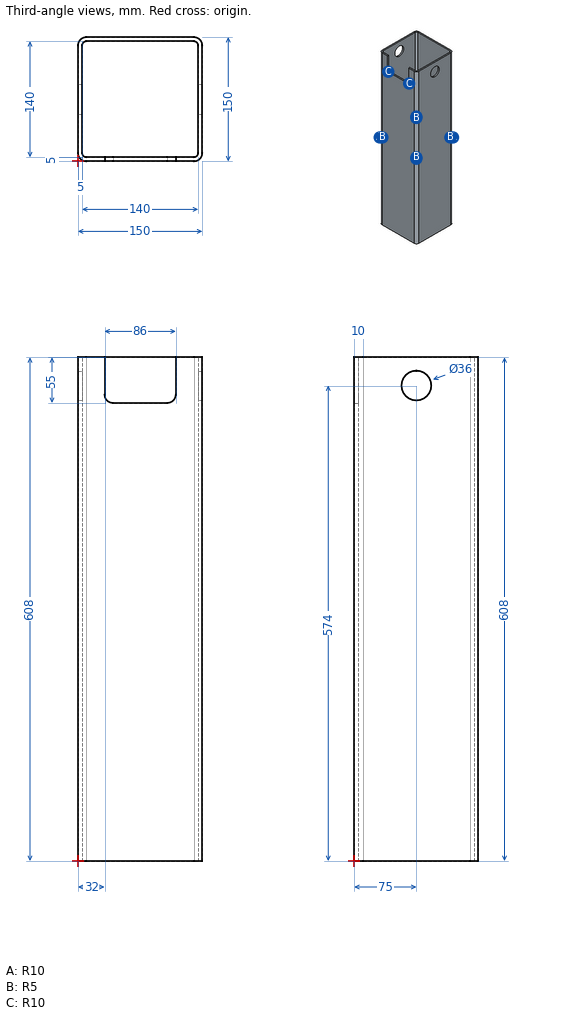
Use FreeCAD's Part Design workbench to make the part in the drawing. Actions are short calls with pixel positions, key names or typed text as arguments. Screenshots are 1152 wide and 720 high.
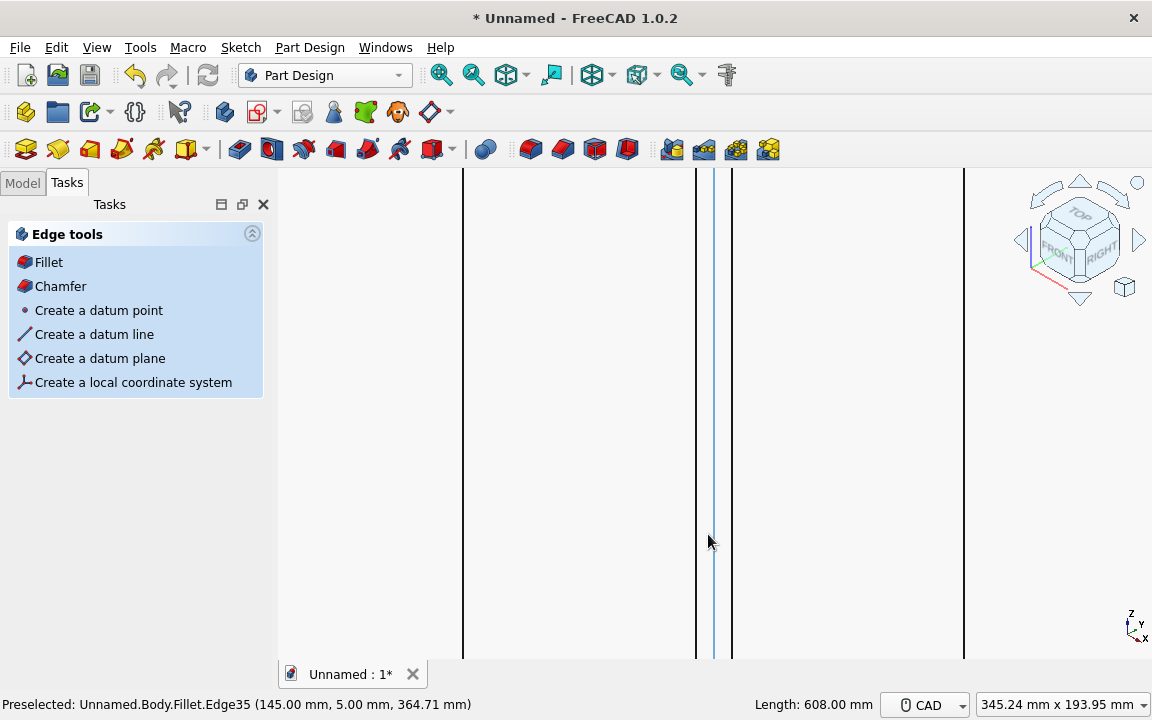
key(v)
key(f)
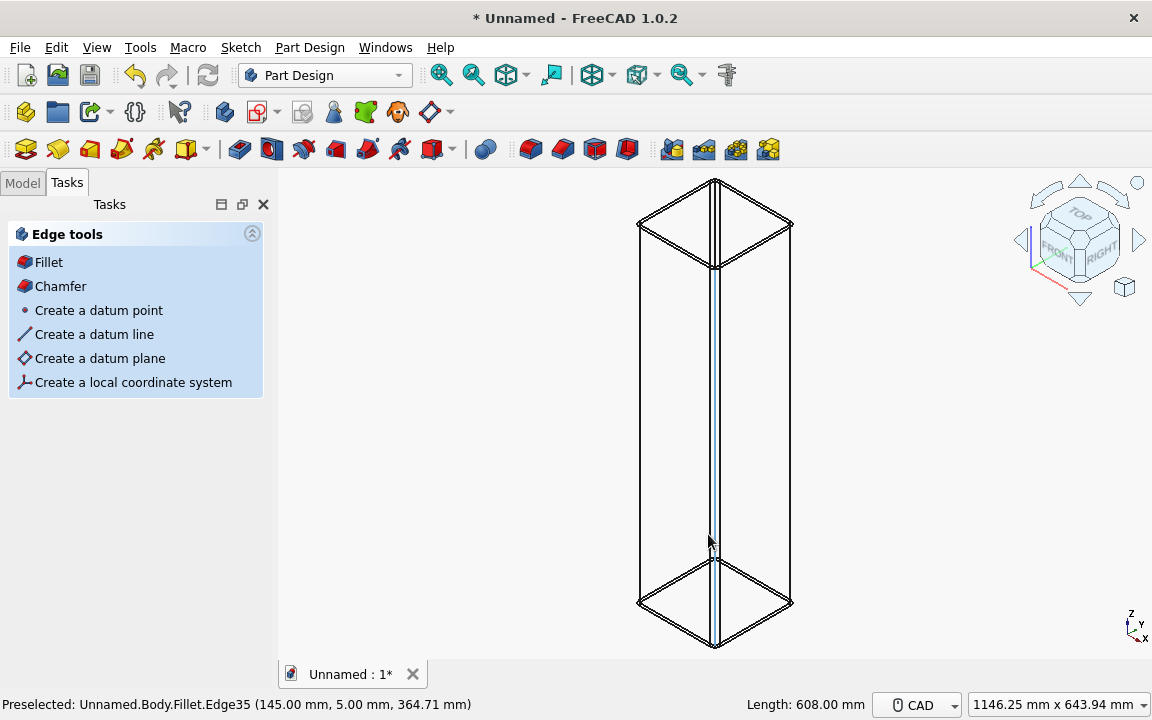
key(2)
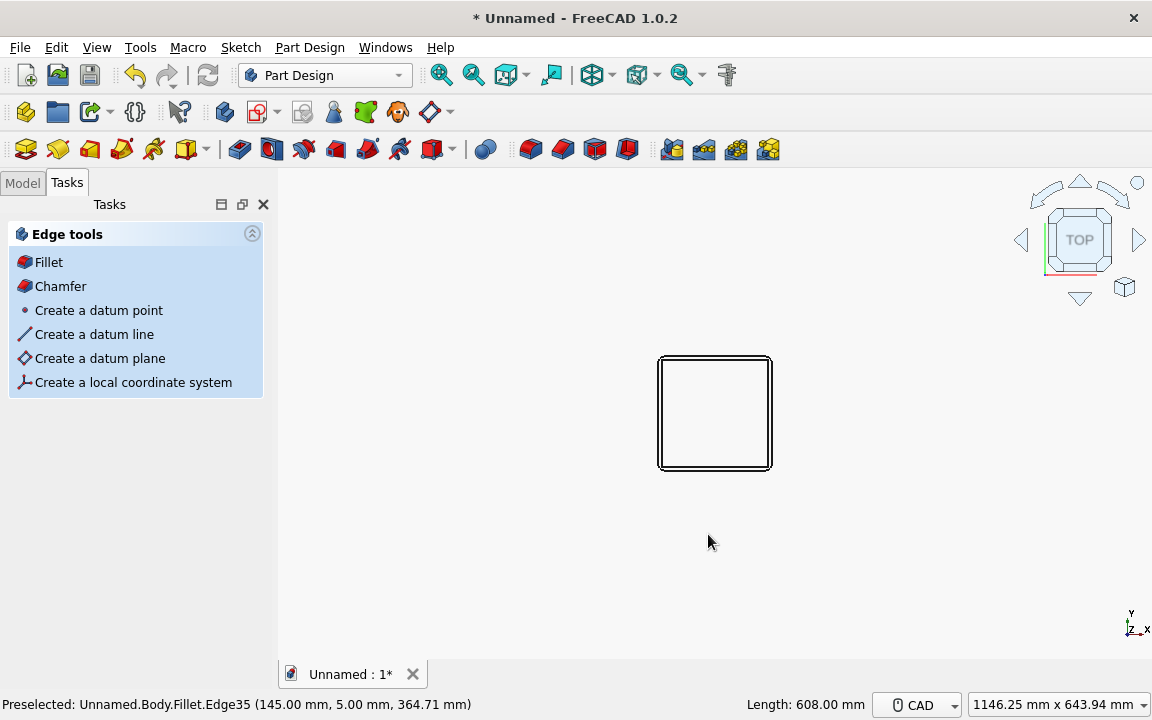
key(v)
key(f)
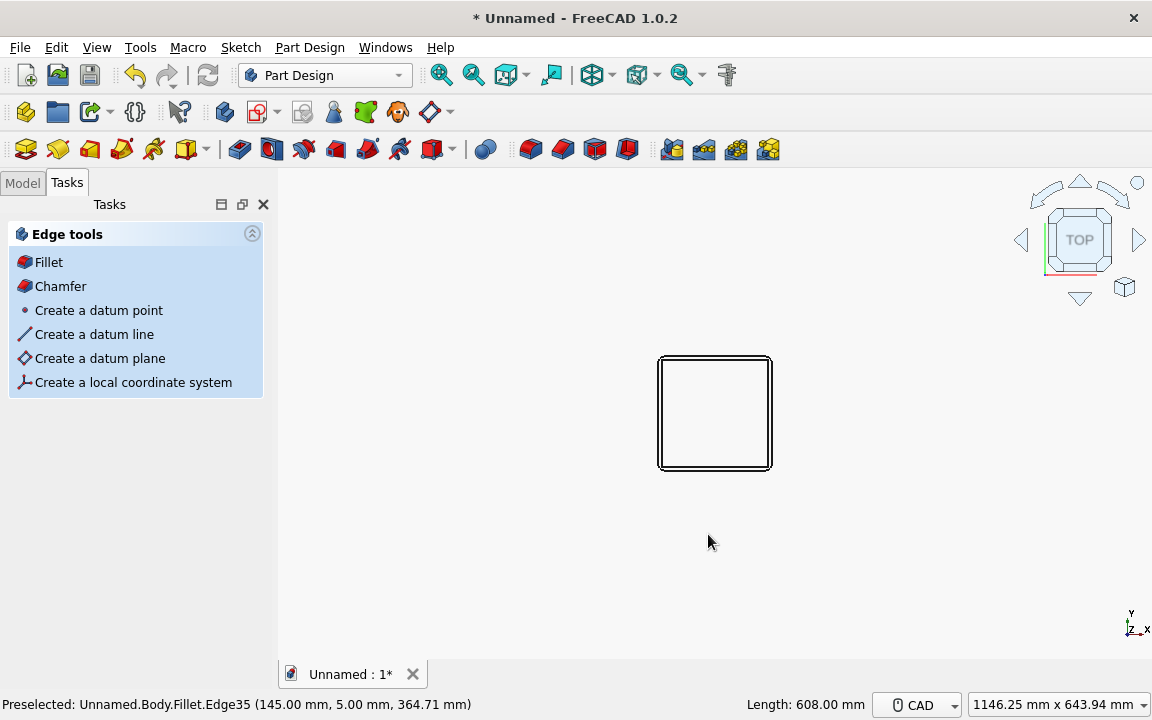
scroll(662, 359, up, 6)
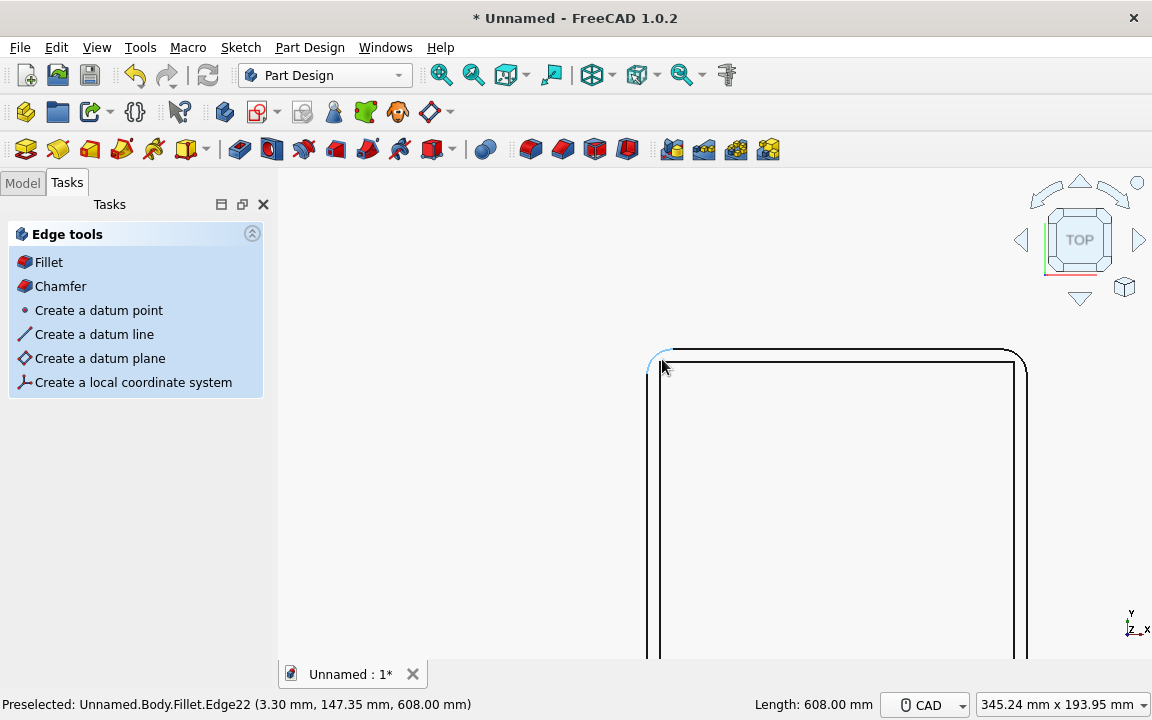
click(442, 76)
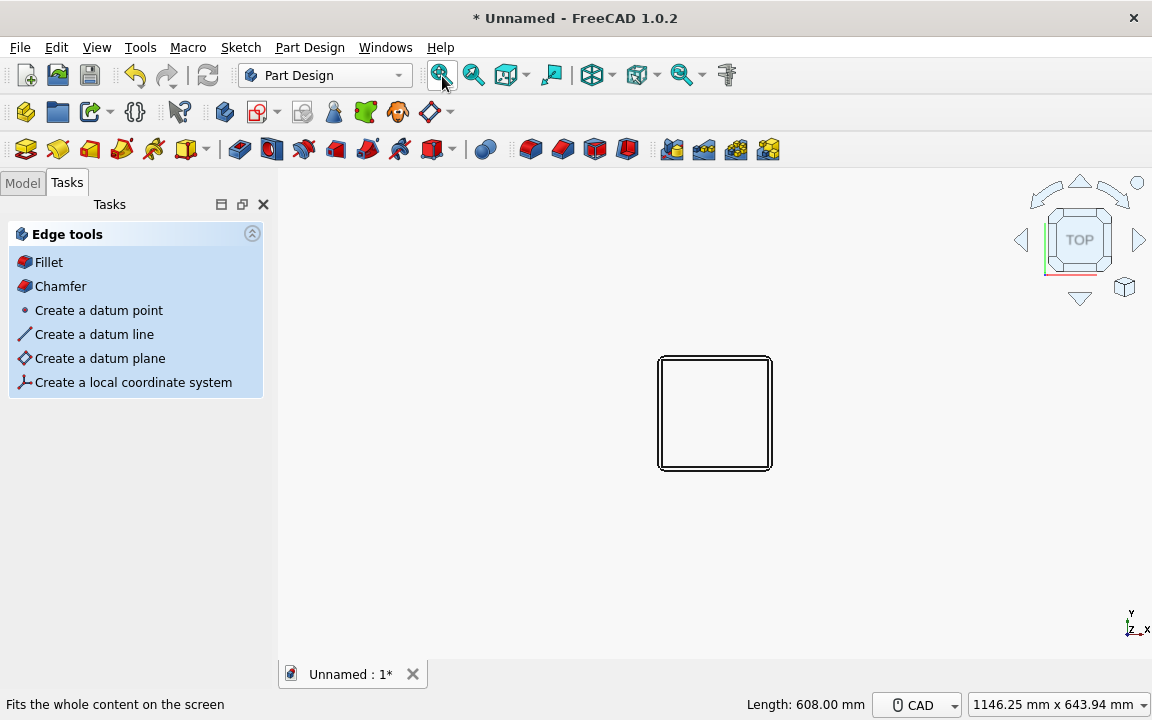
key(1)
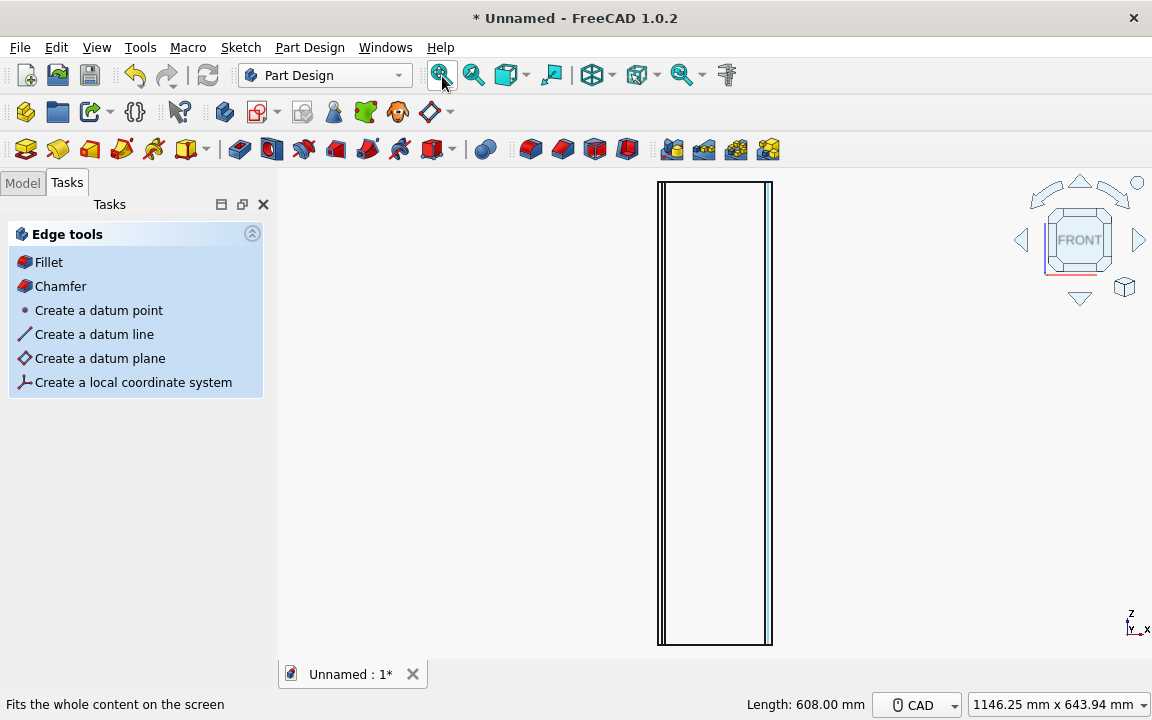
scroll(662, 413, up, 6)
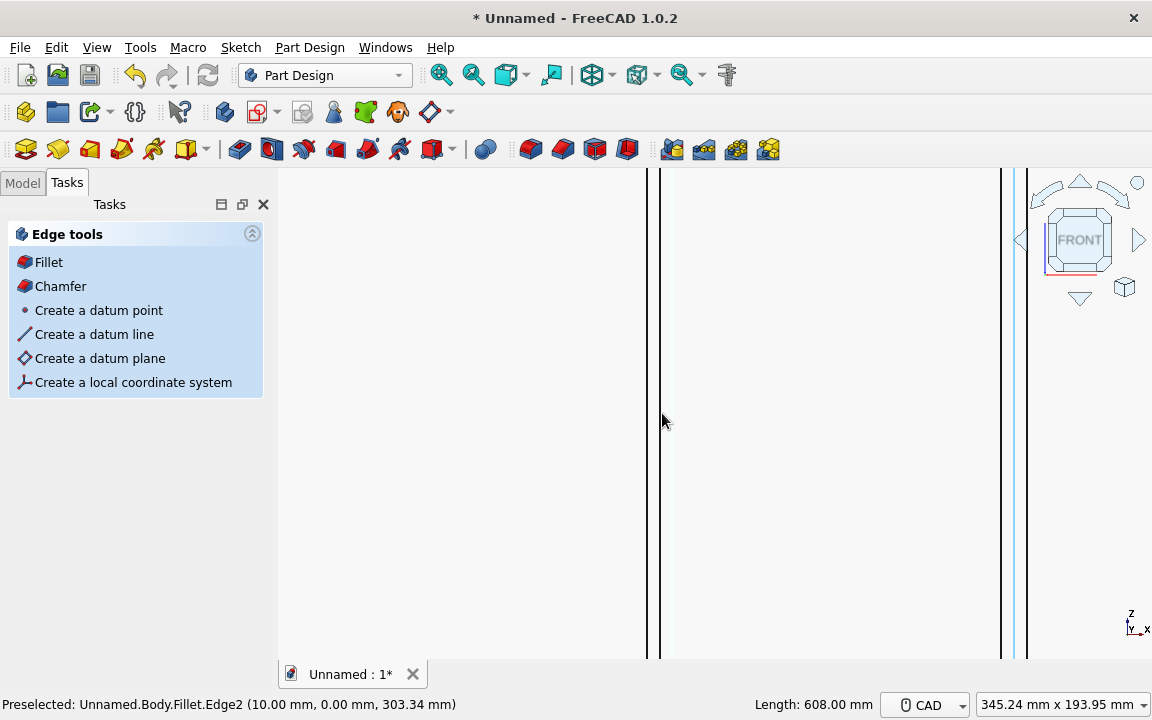
click(660, 413, ctrl)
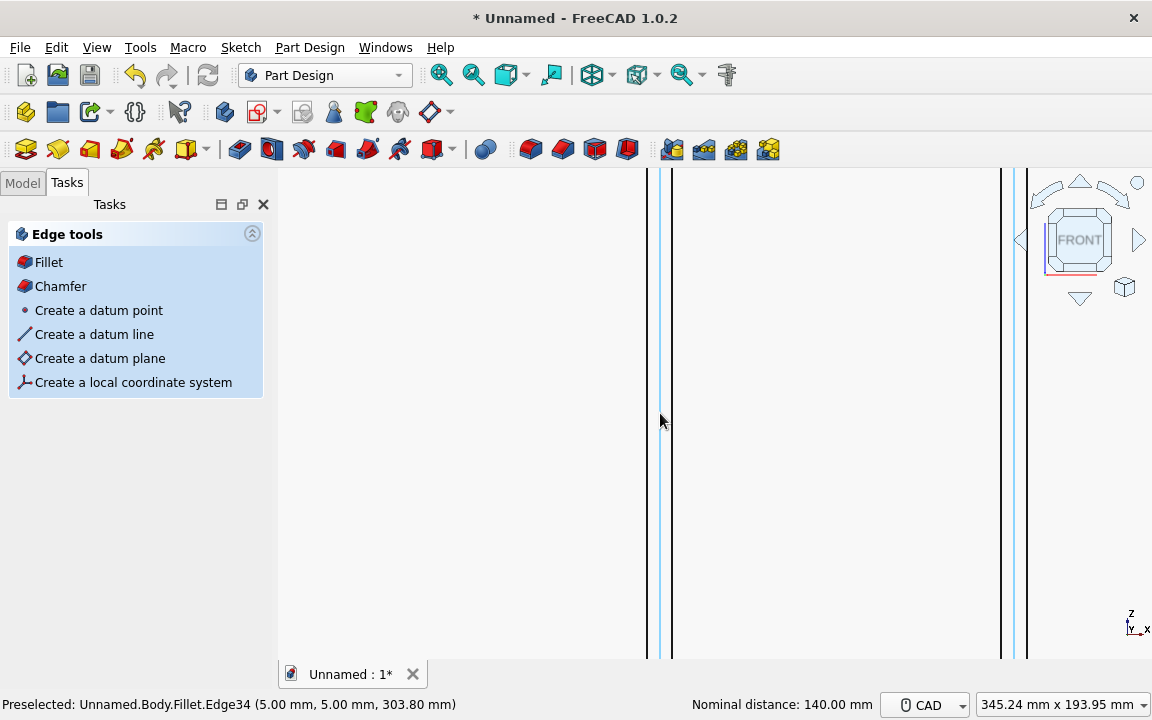
key(v)
key(f)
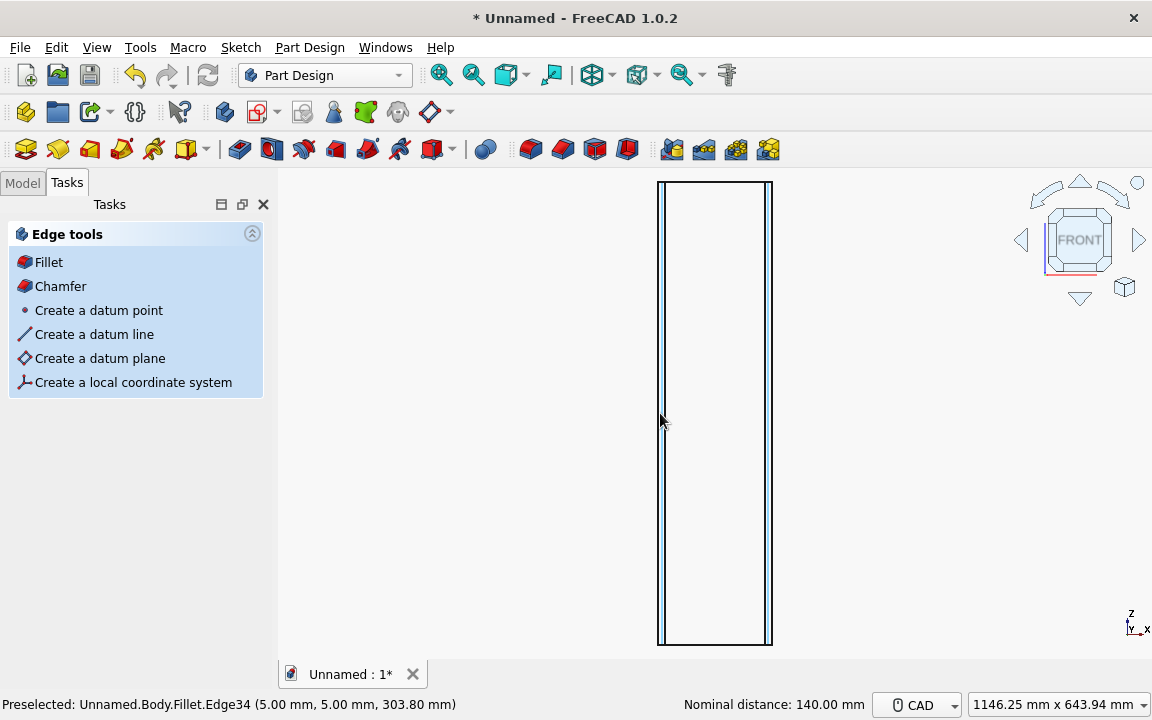
key(3)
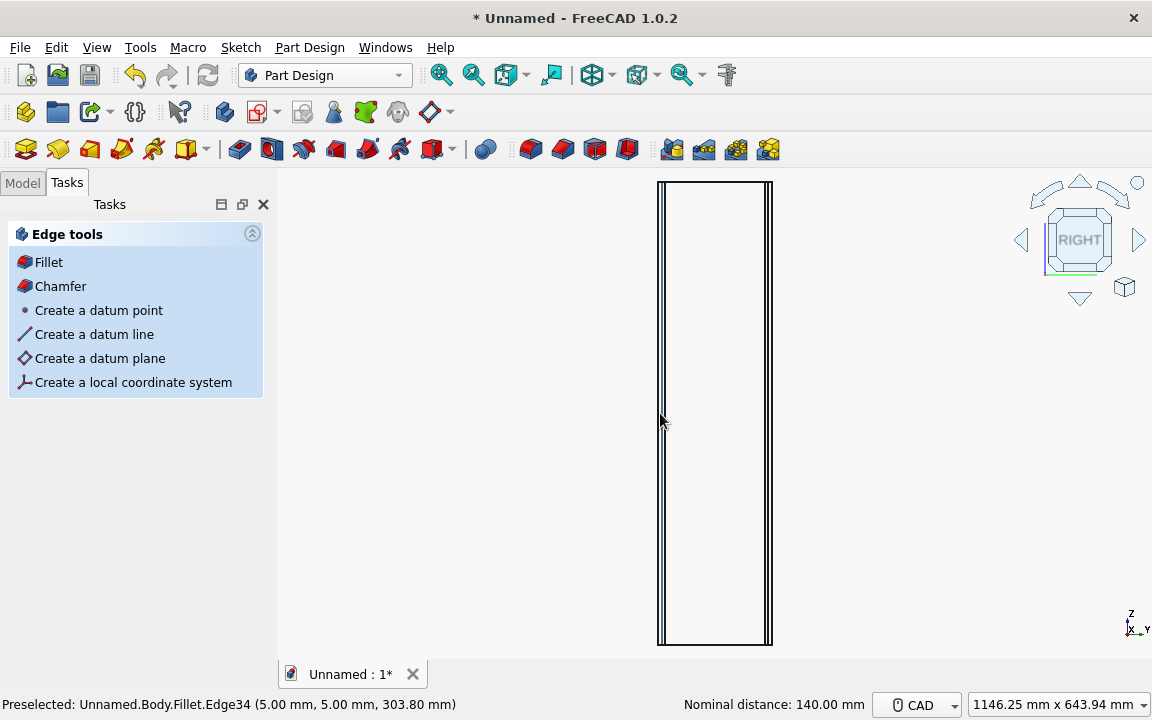
scroll(768, 412, up, 6)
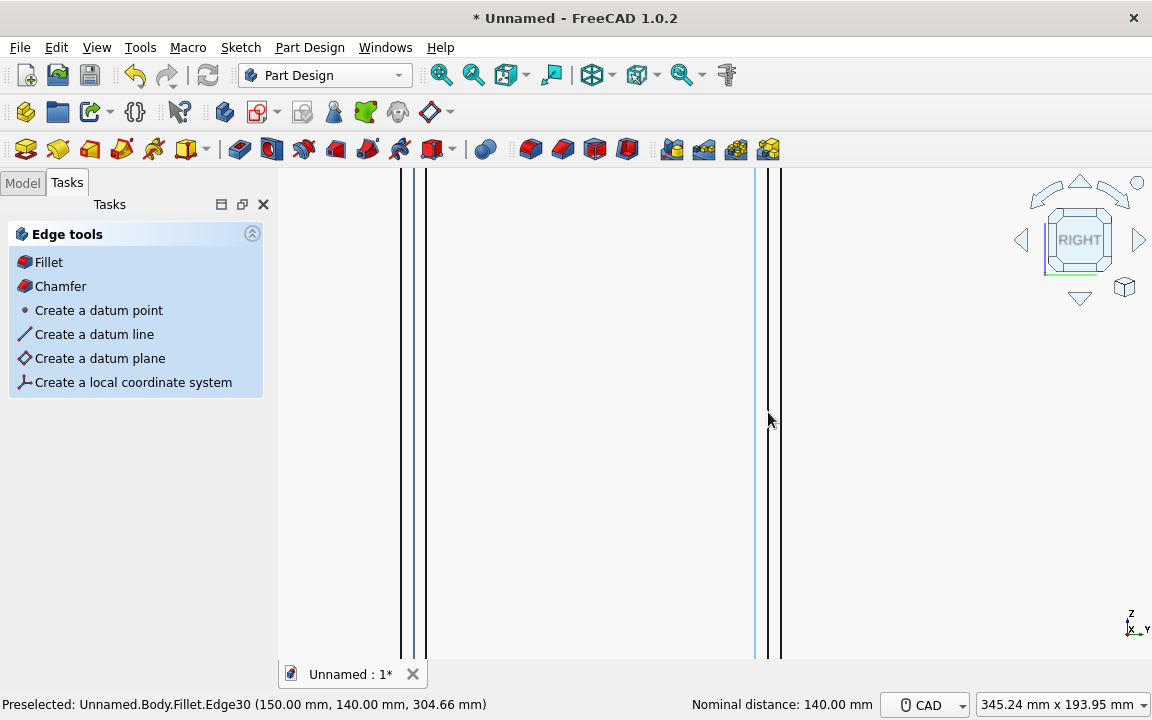
click(768, 415, ctrl)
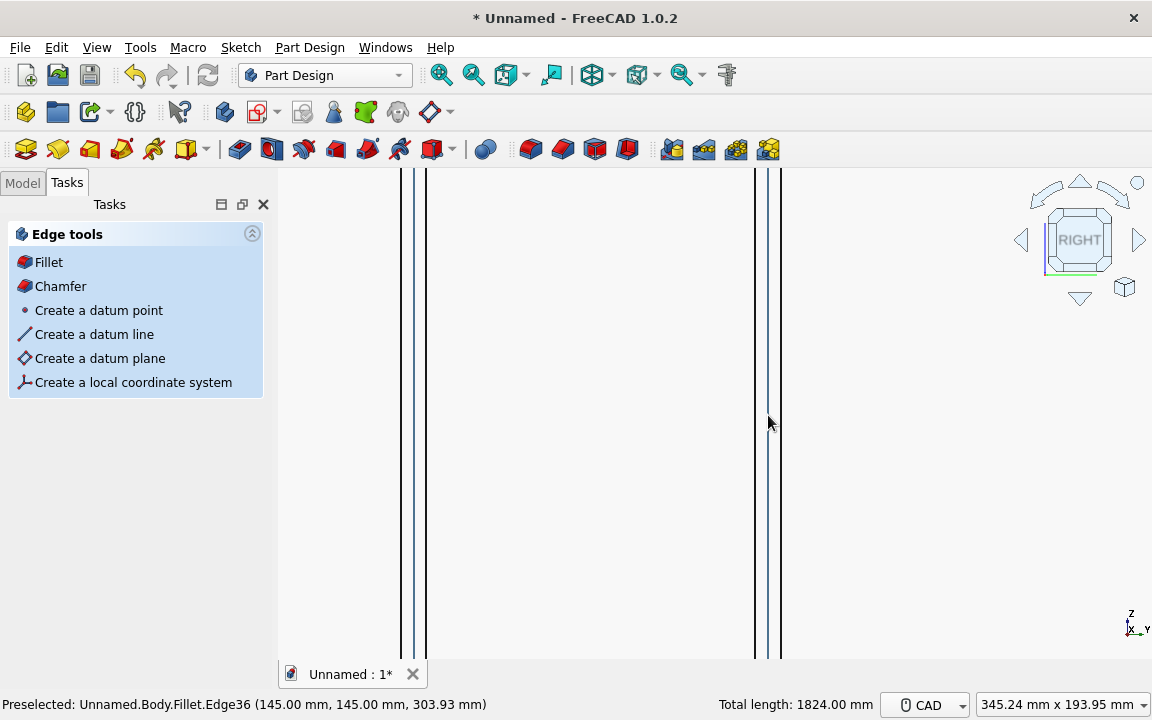
key(v)
key(f)